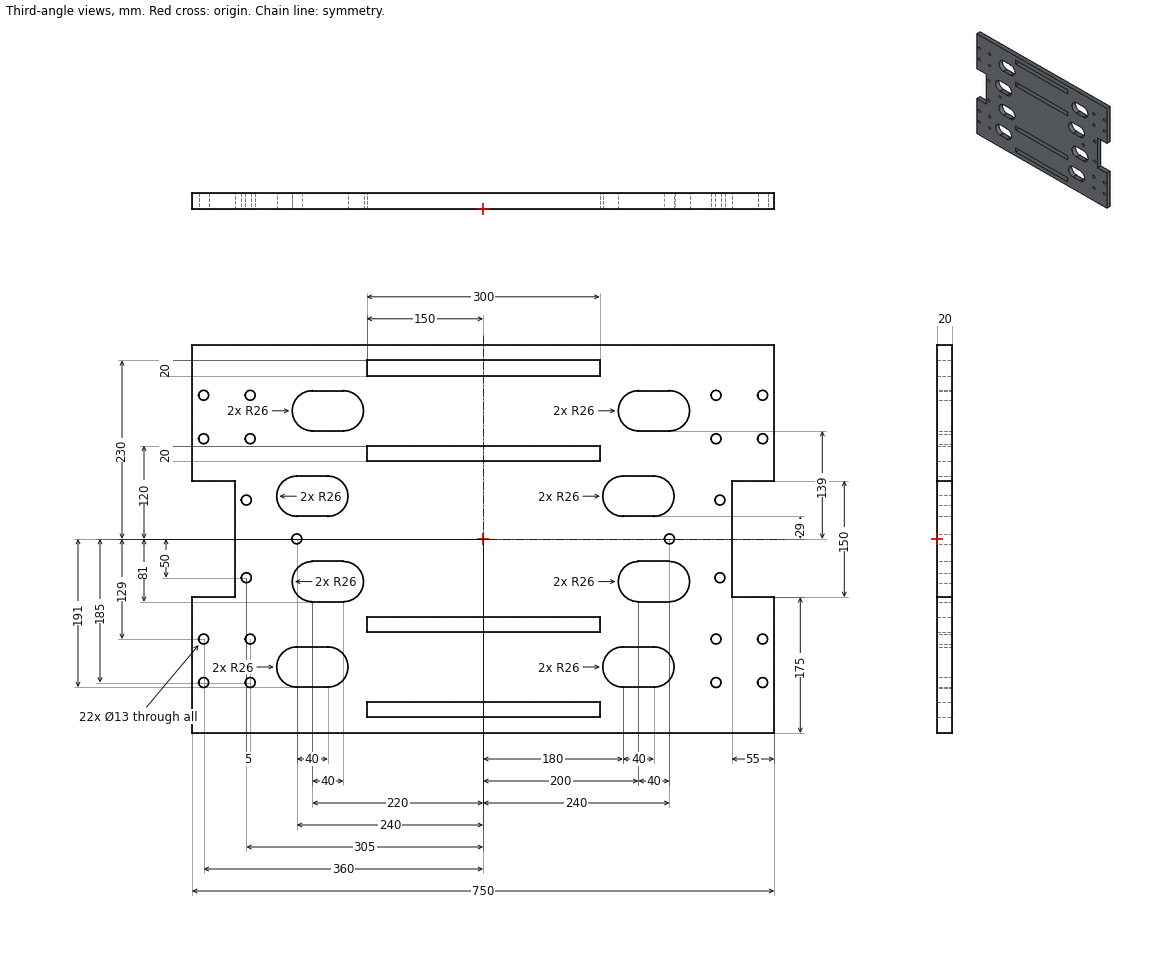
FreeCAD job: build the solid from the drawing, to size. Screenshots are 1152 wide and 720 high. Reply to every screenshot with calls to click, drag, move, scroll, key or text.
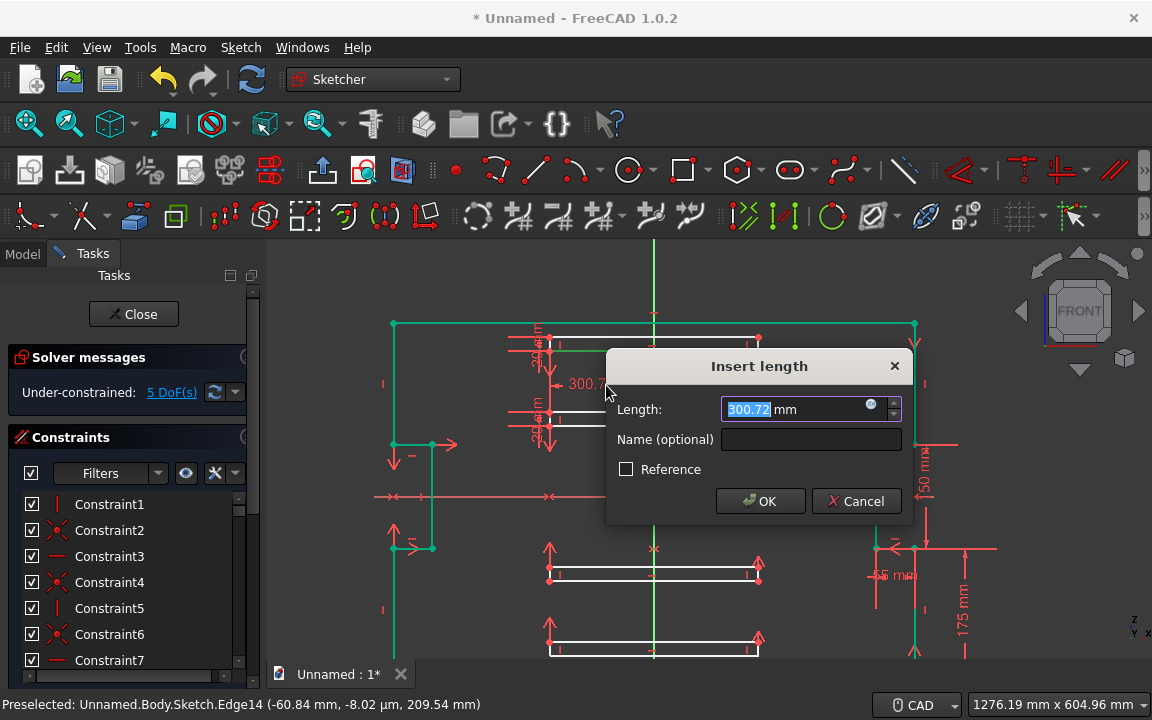
text(300)
key(Return)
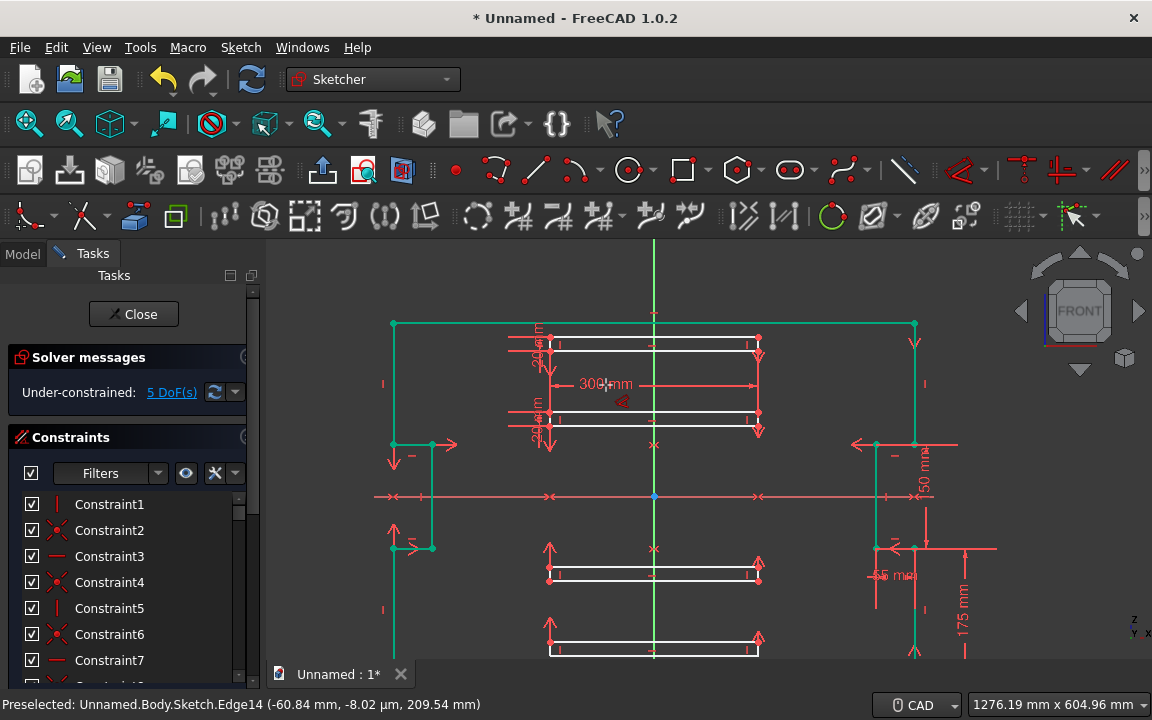
click(612, 426)
click(702, 392)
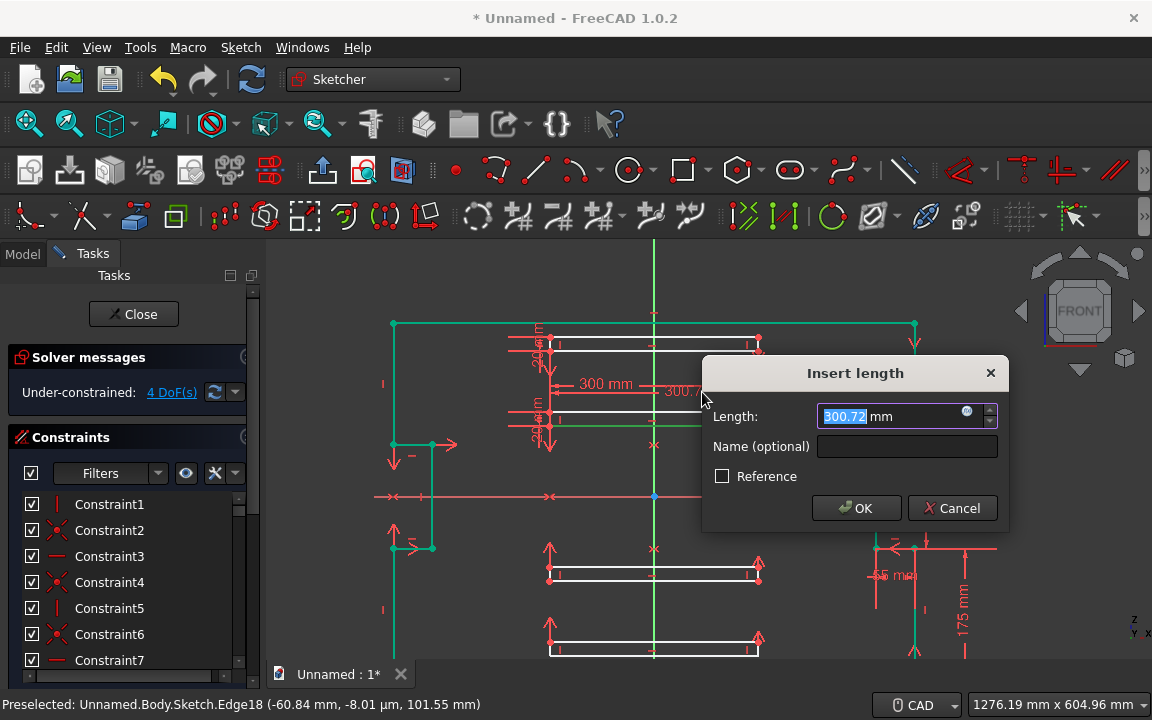
text(300)
key(Return)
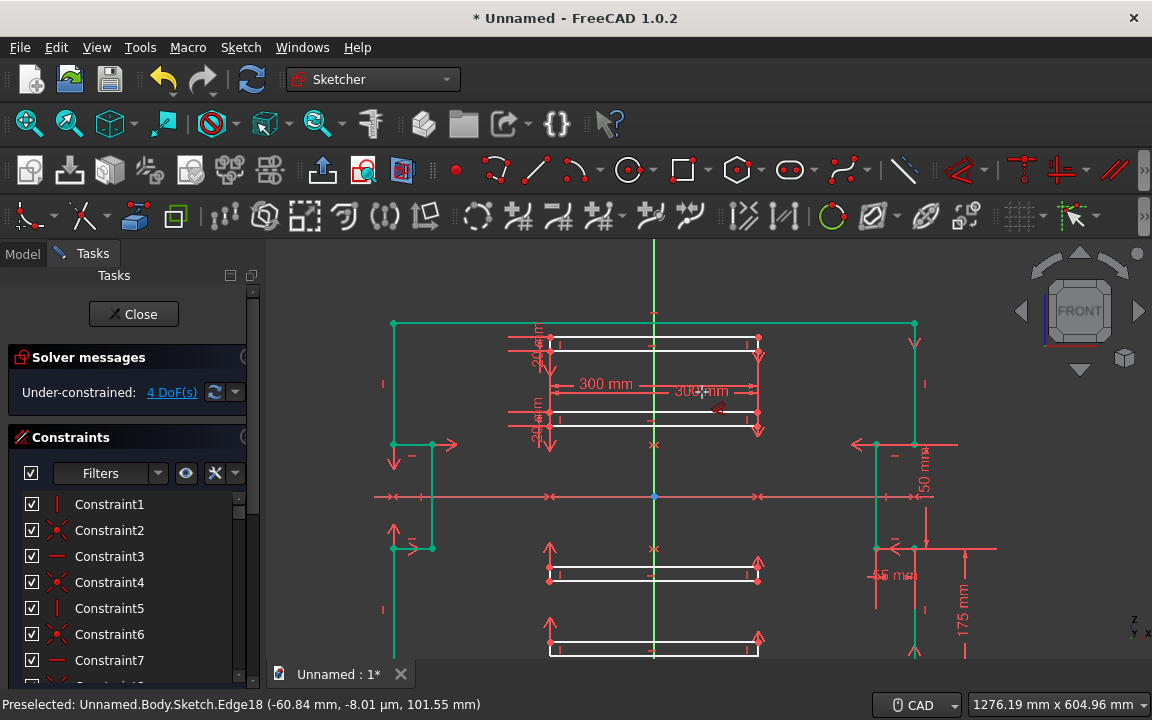
click(550, 337)
click(602, 303)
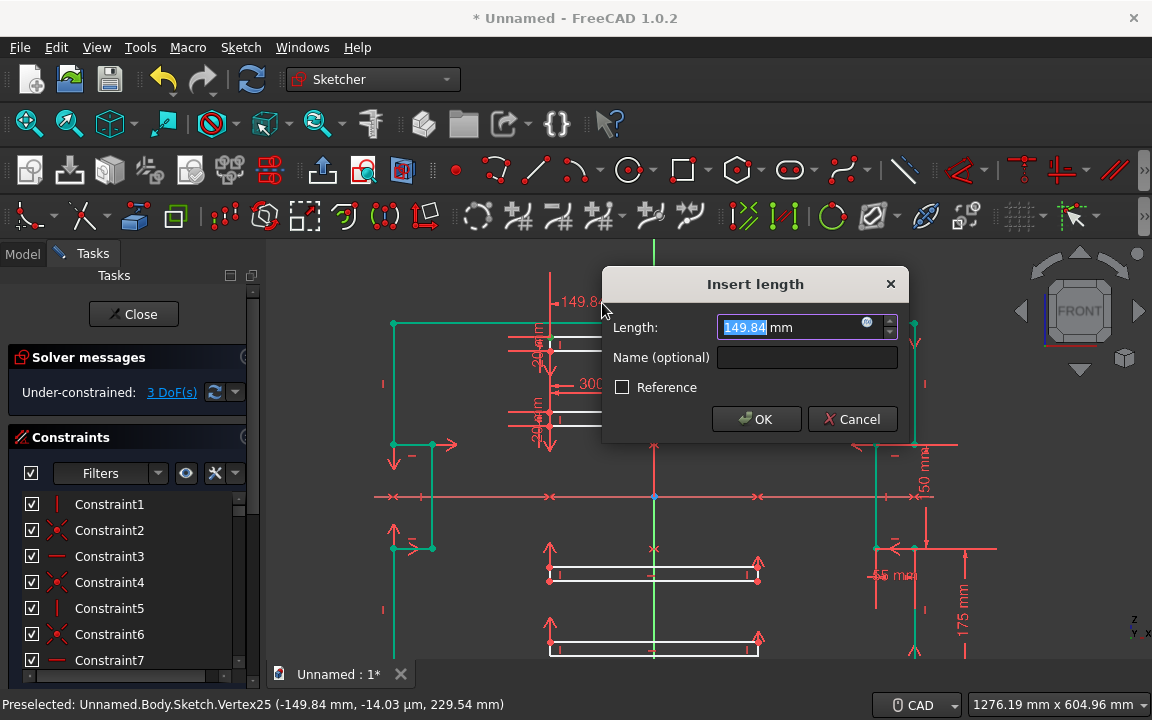
text(150)
key(Return)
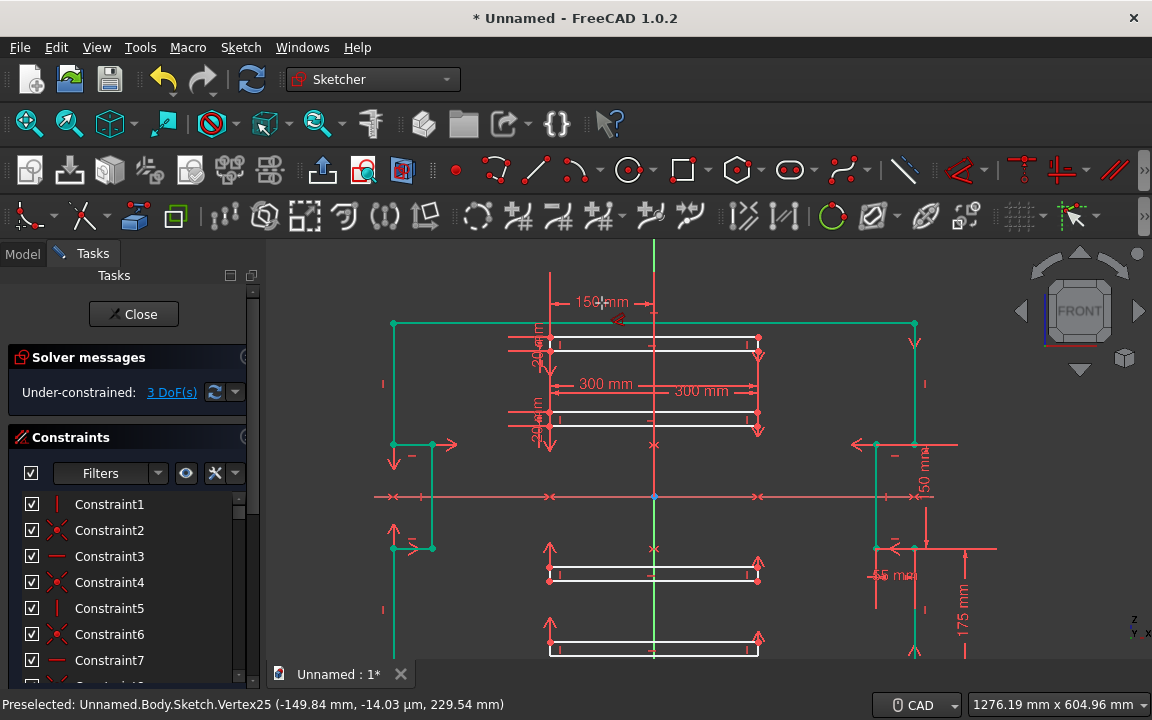
click(550, 337)
click(516, 380)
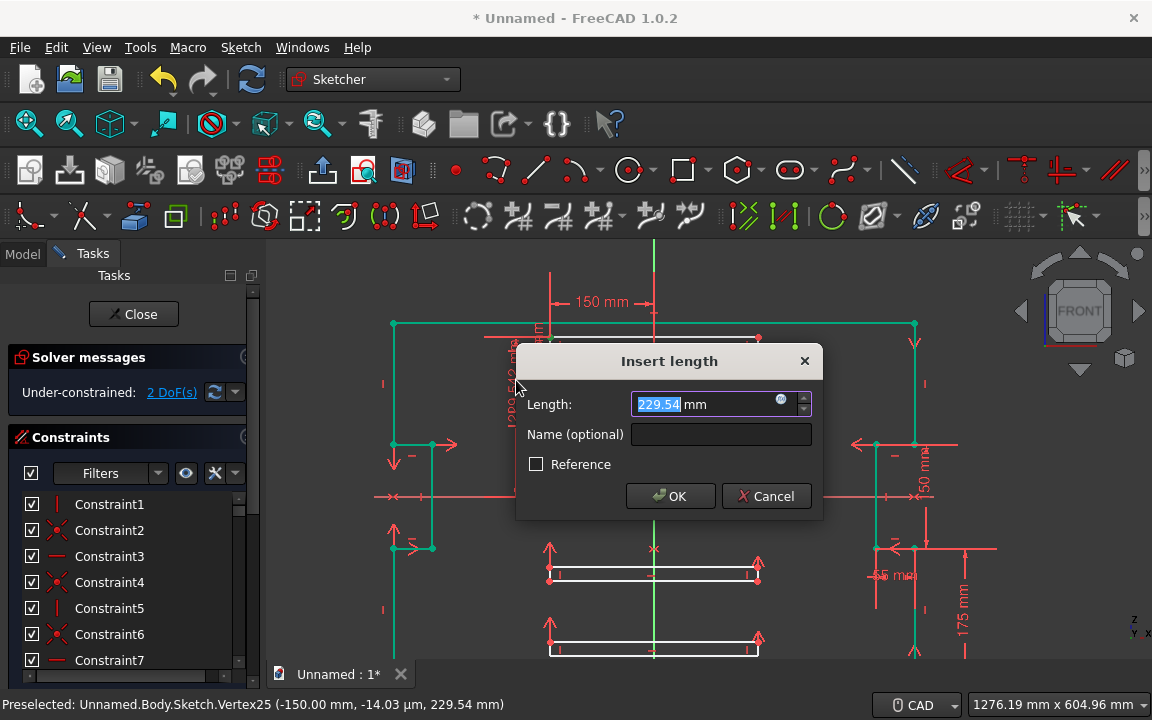
text(230)
key(Return)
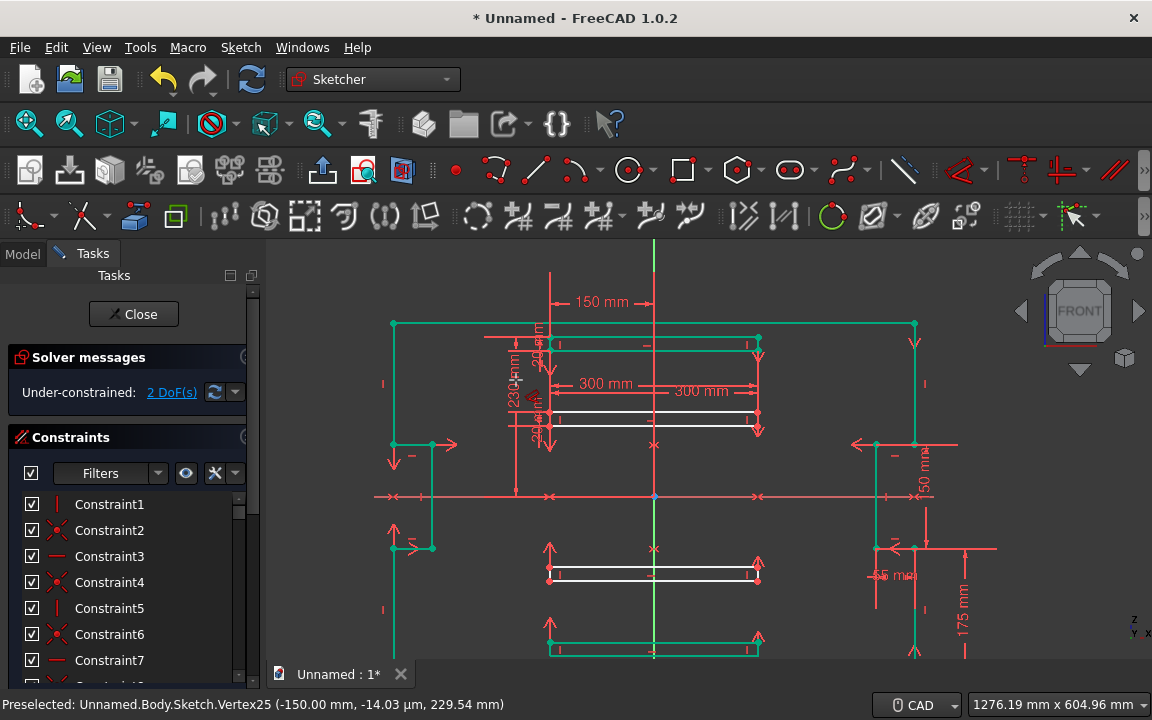
click(550, 412)
click(602, 531)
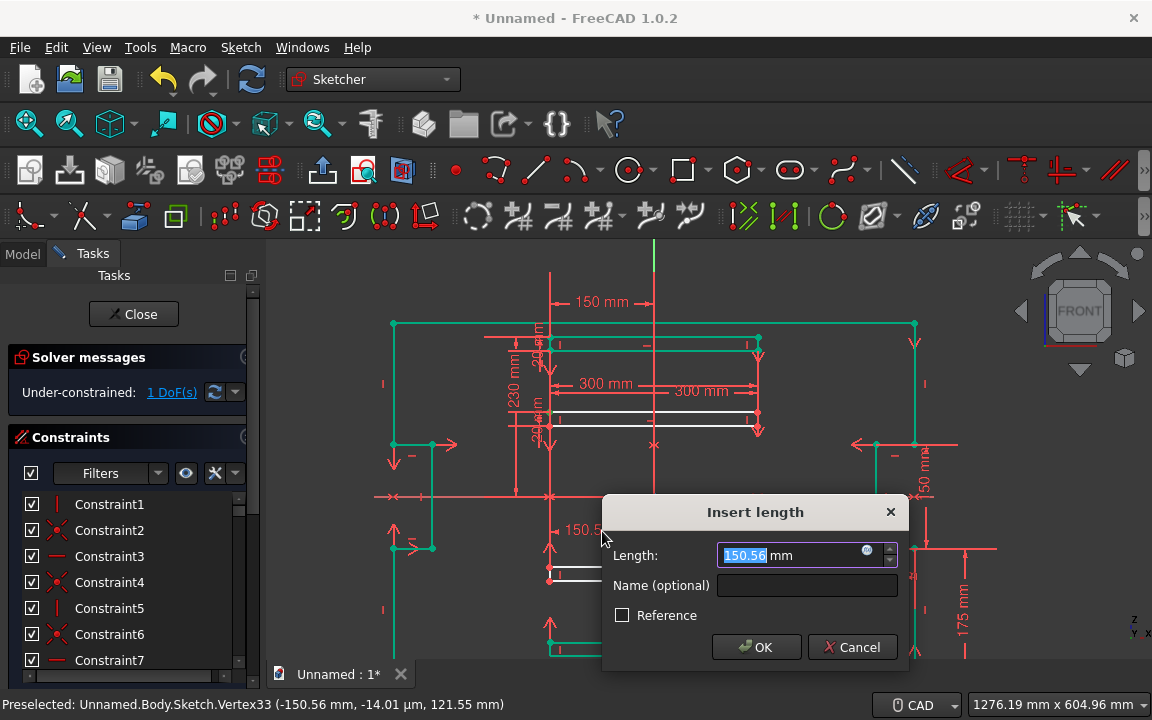
text(150)
key(Return)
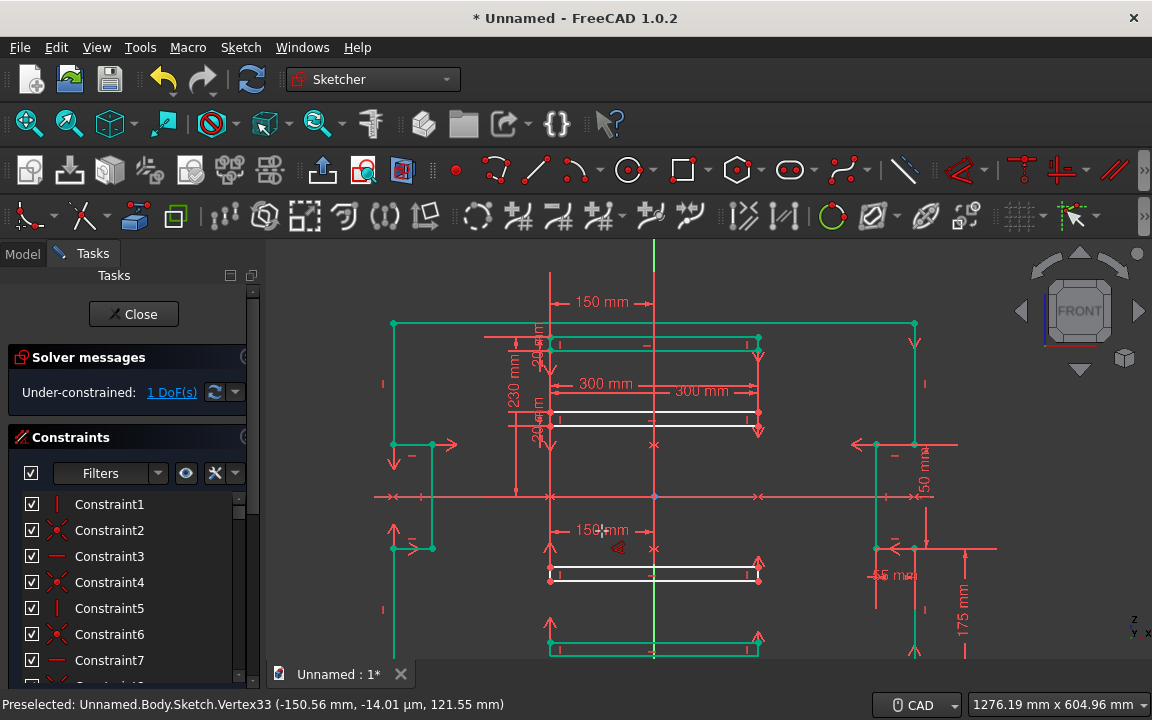
click(550, 412)
click(516, 455)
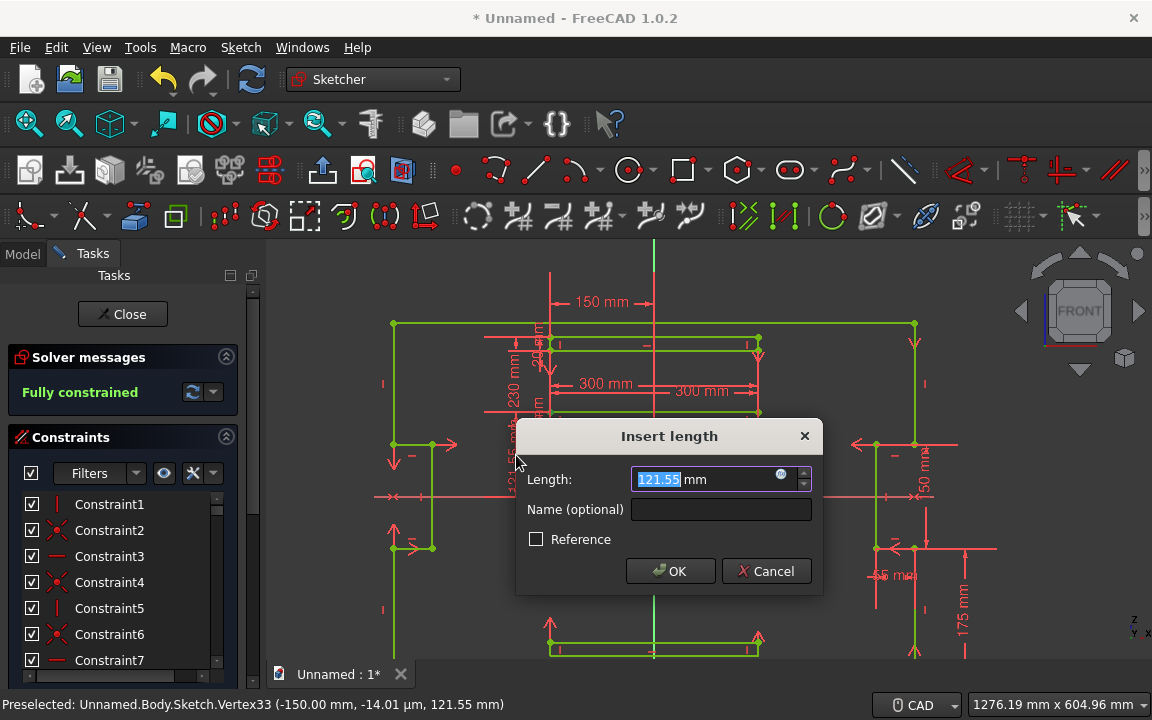
text(120)
key(Return)
key(Escape)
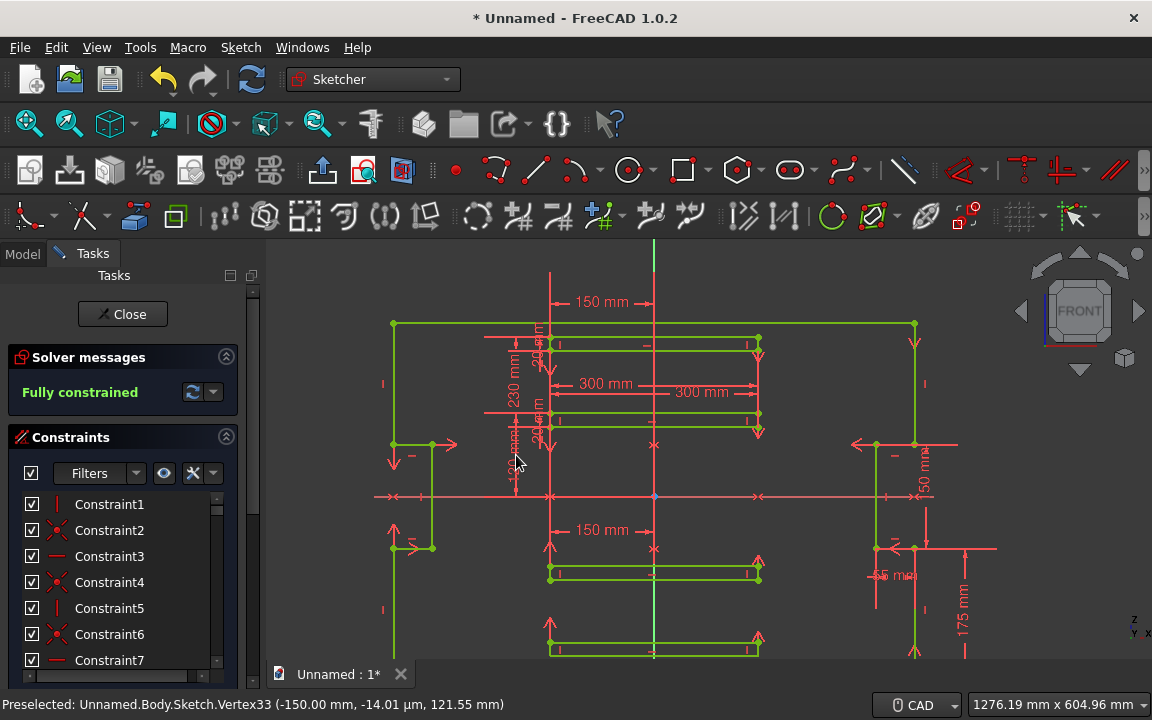
click(123, 314)